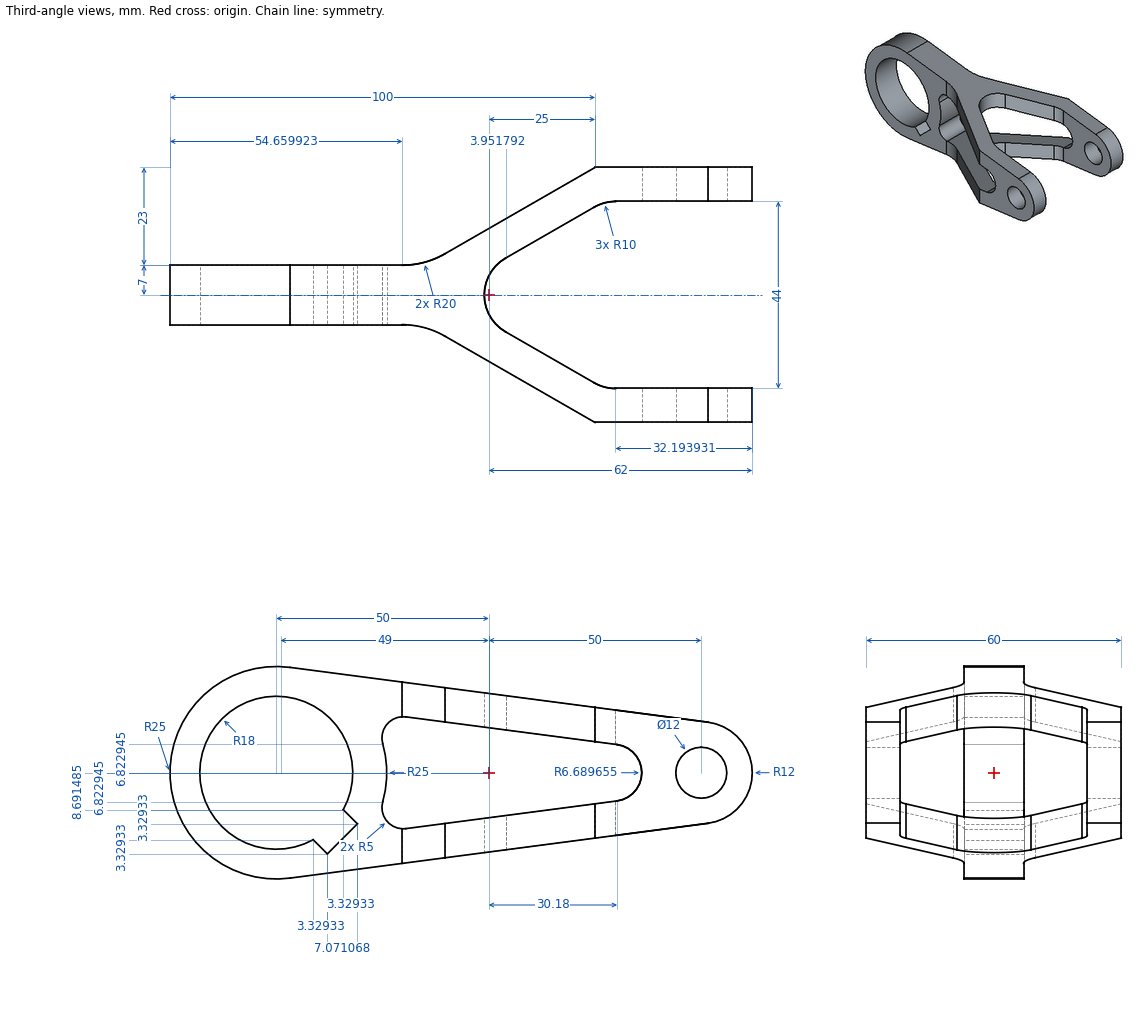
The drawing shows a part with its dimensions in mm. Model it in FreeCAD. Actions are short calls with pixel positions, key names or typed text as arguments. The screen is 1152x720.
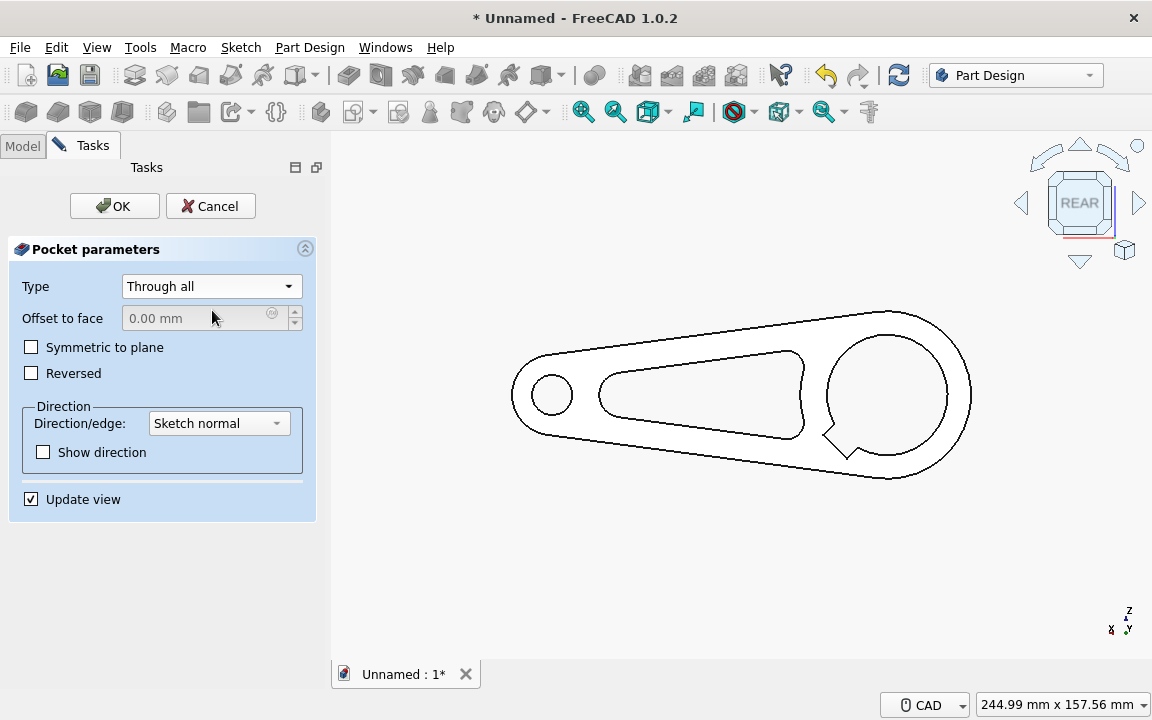
click(115, 206)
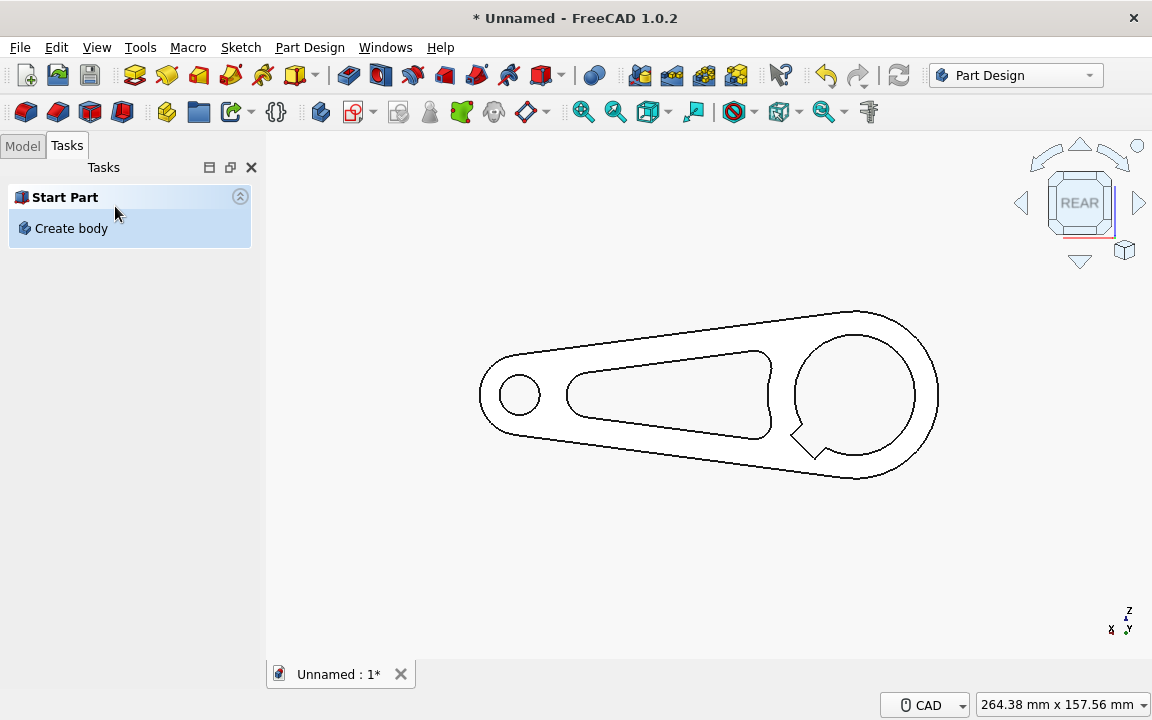
click(354, 112)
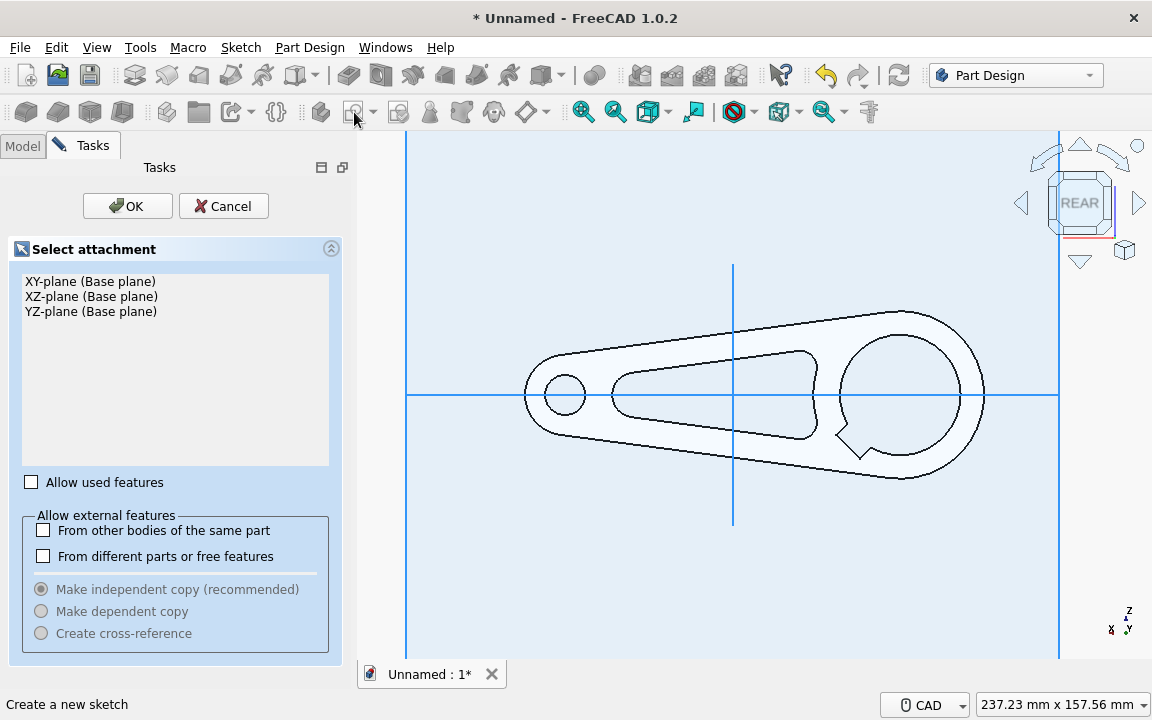
click(82, 282)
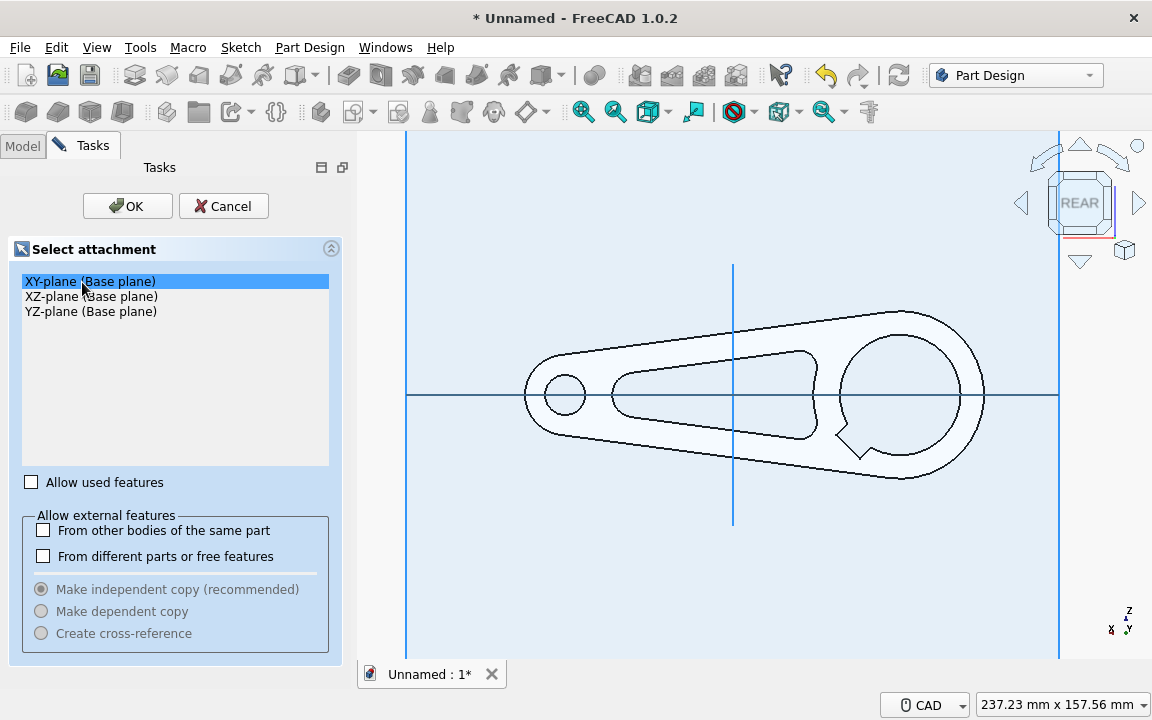
click(128, 206)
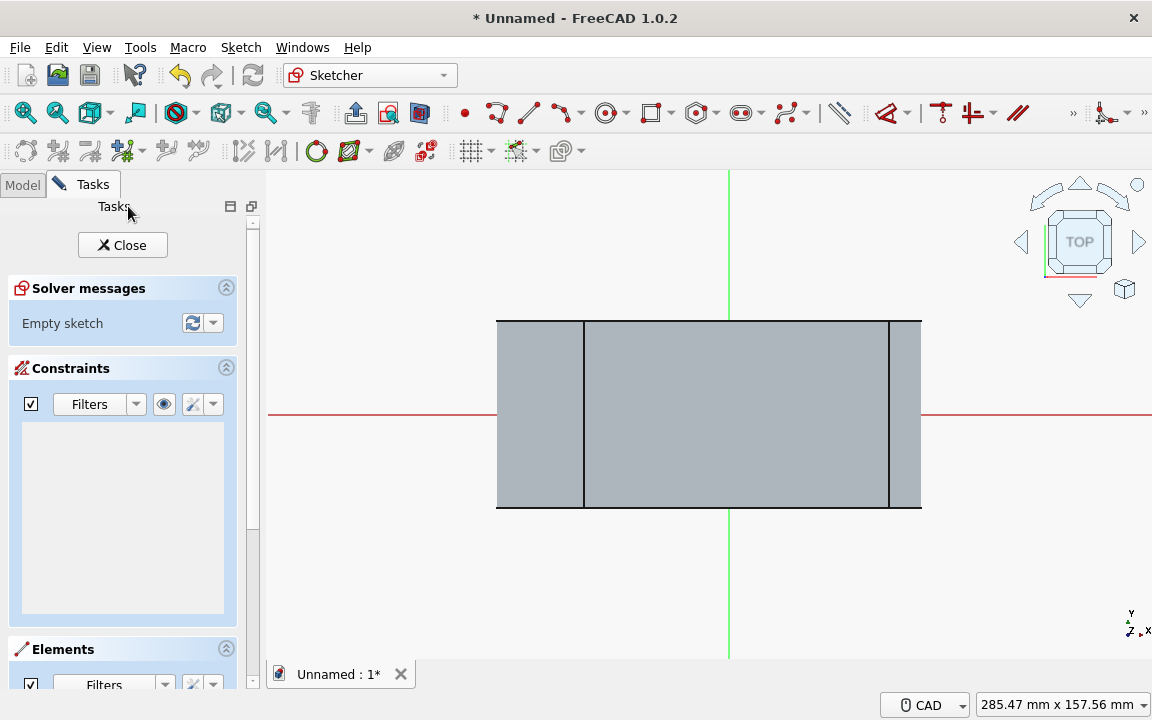
click(420, 114)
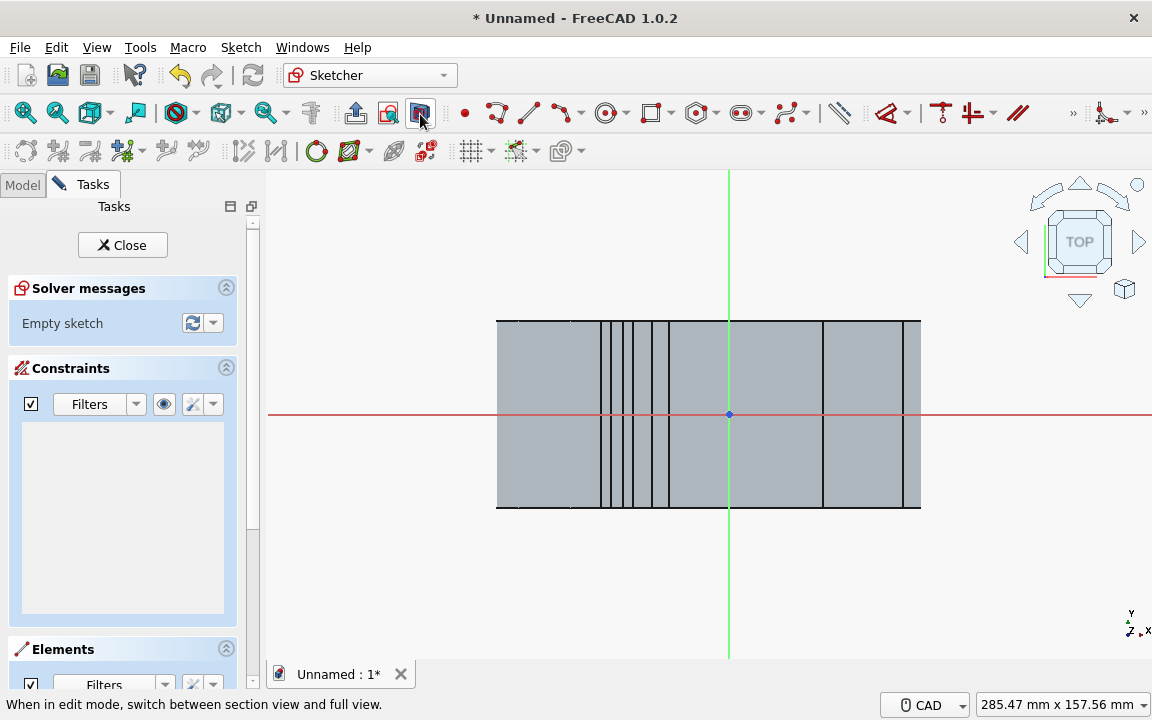
scroll(674, 414, up, 2)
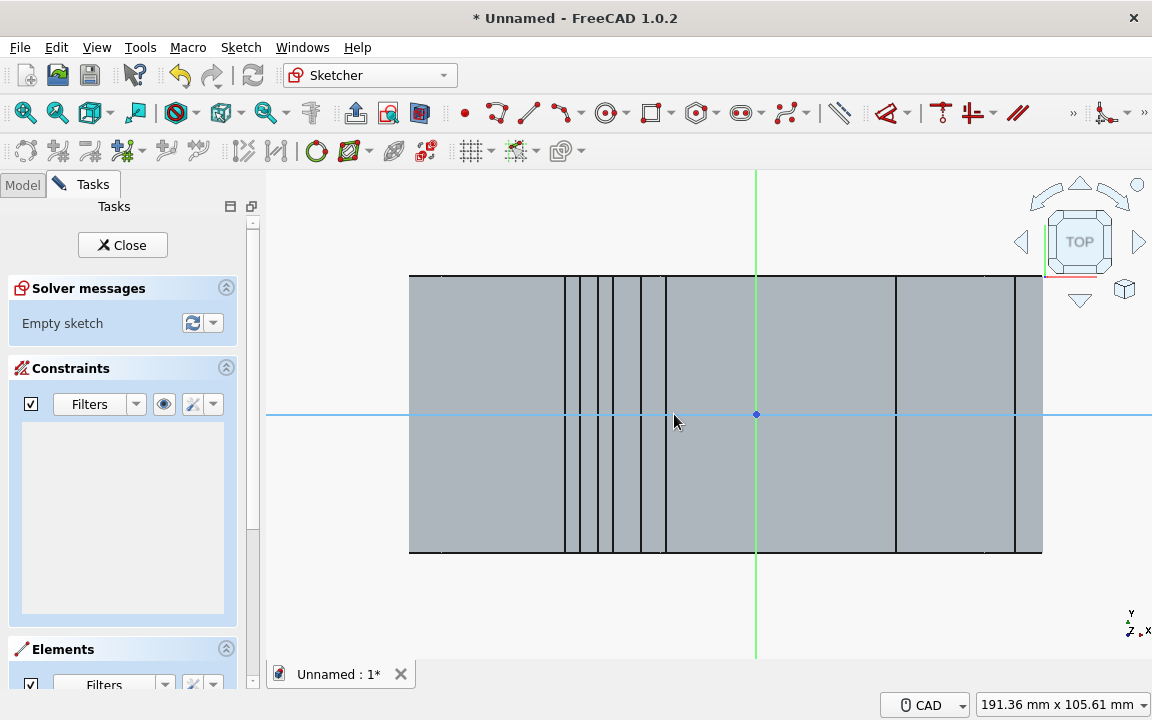
click(498, 114)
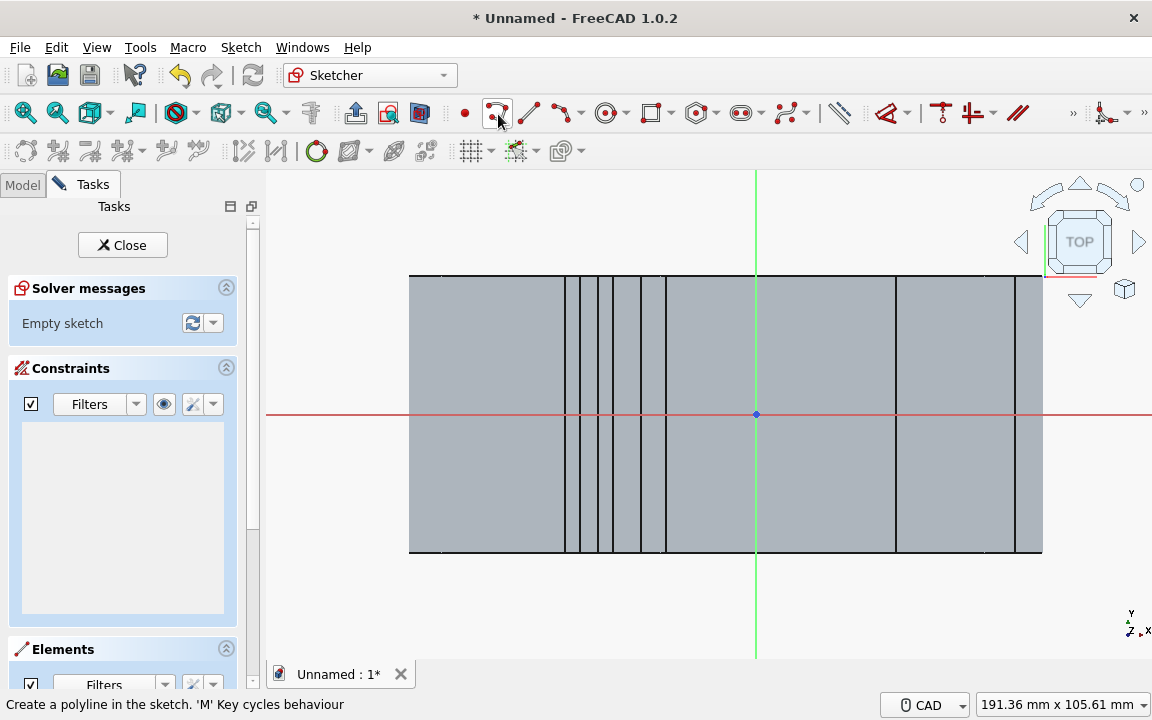
click(708, 370)
click(872, 276)
click(409, 276)
click(409, 382)
click(662, 382)
right_click(662, 382)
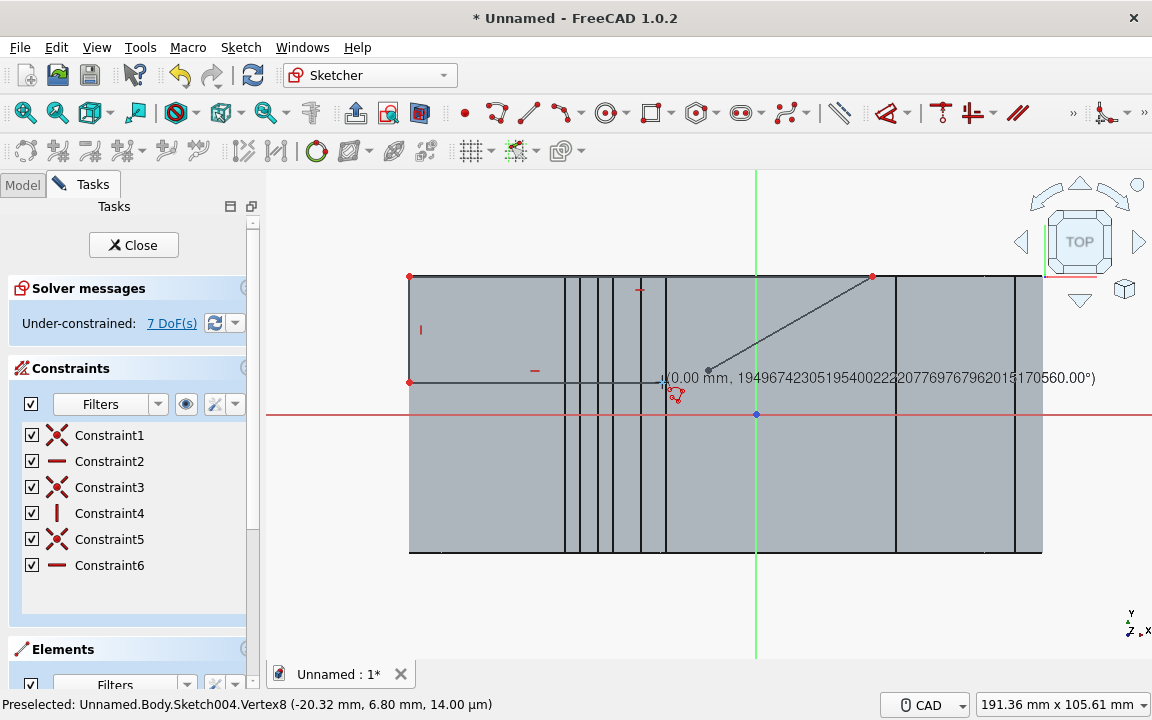
click(562, 114)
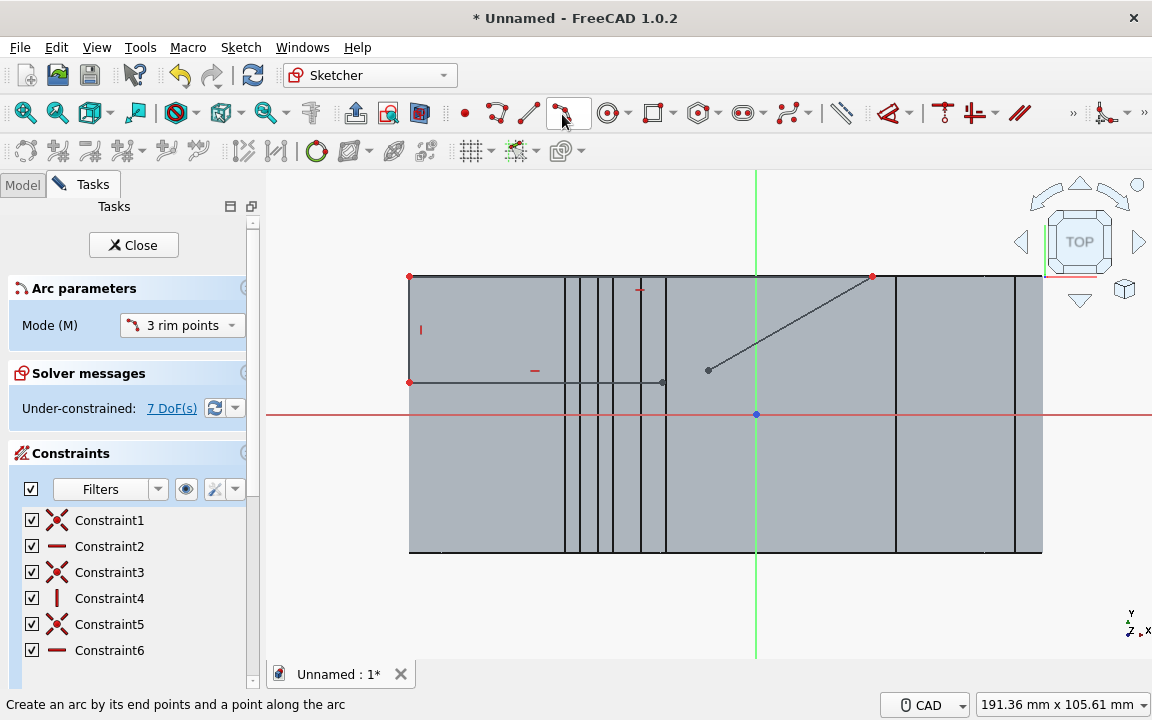
click(662, 383)
click(708, 371)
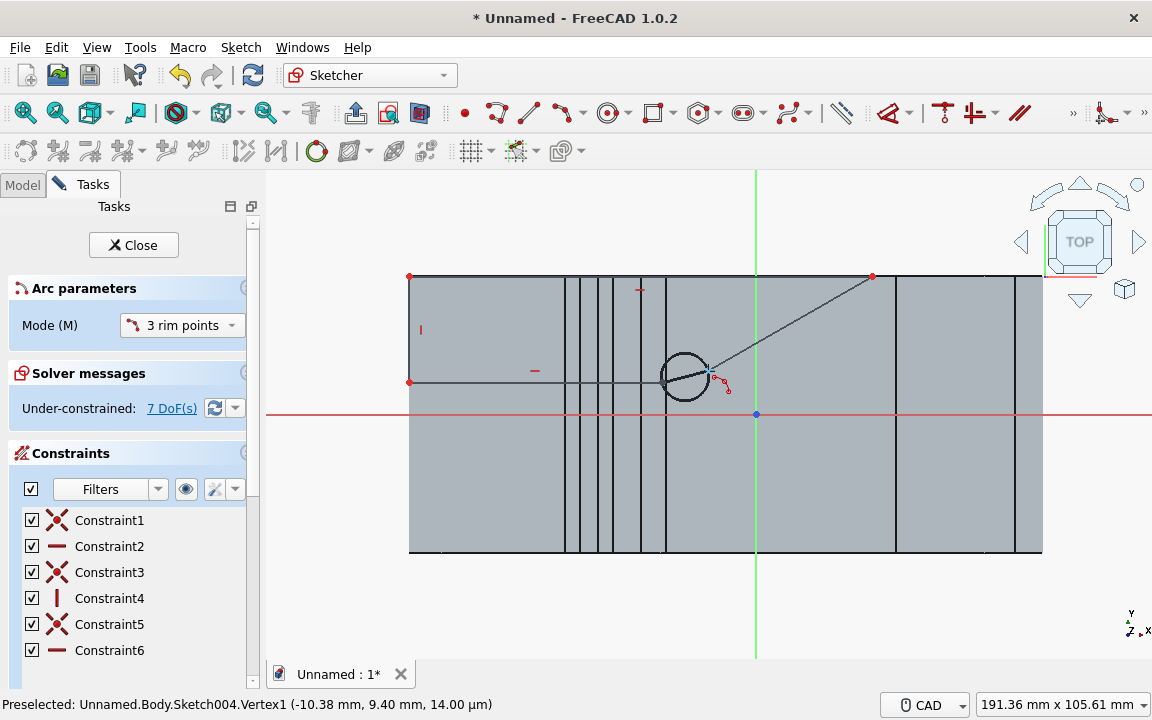
scroll(686, 379, up, 9)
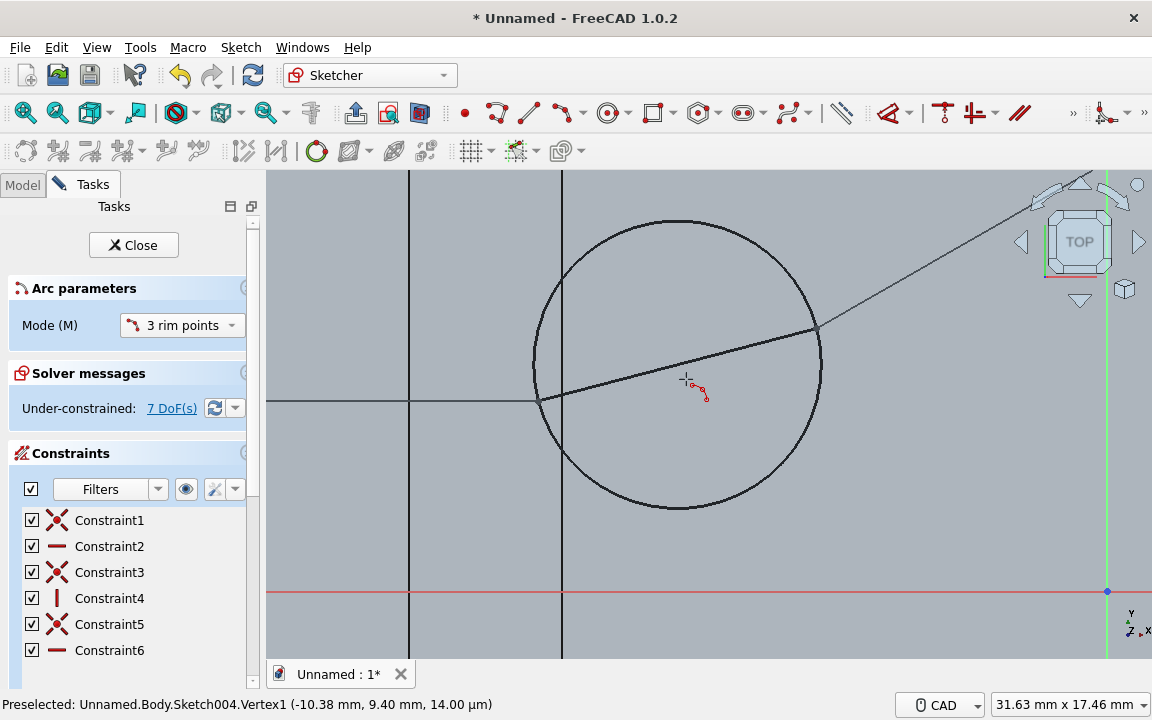
click(682, 377)